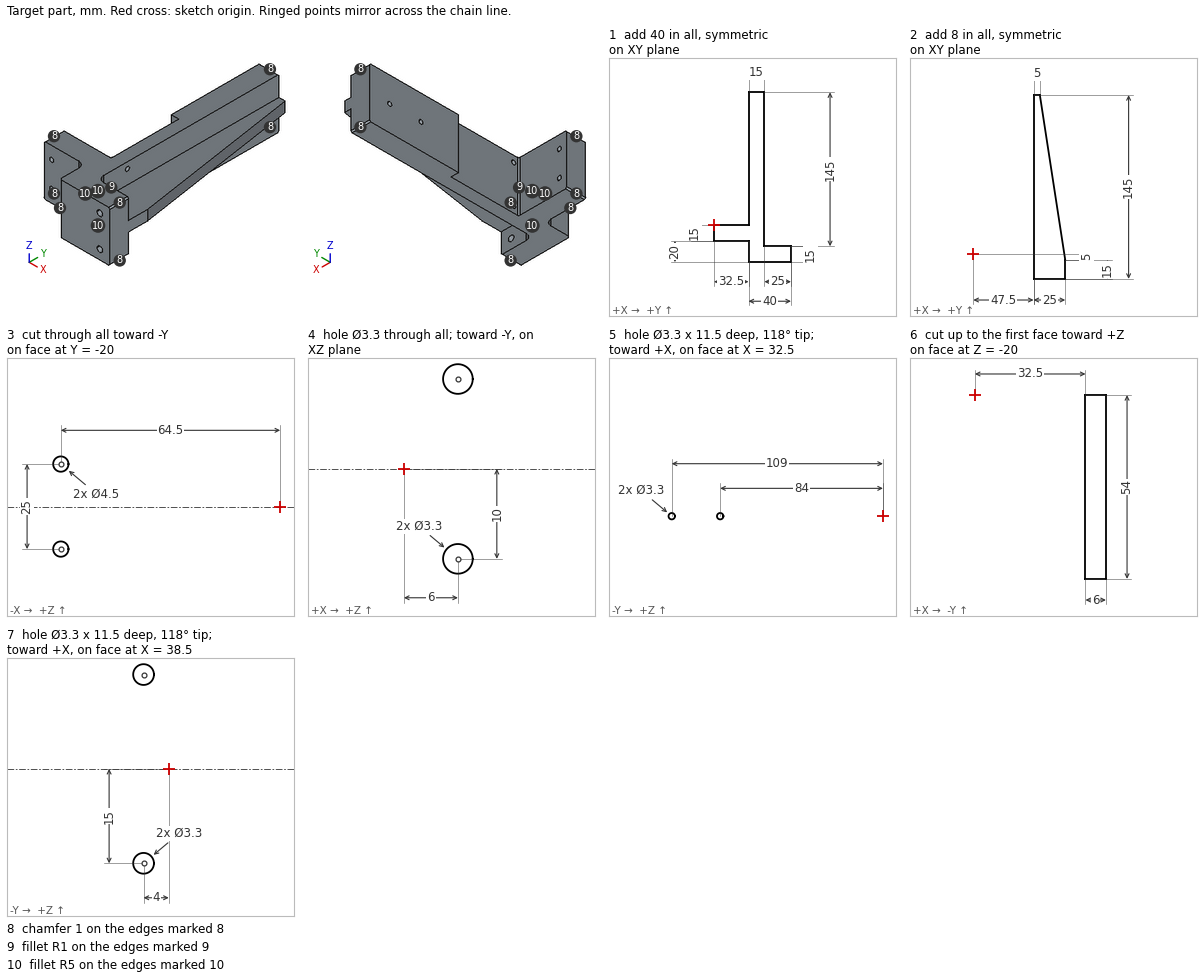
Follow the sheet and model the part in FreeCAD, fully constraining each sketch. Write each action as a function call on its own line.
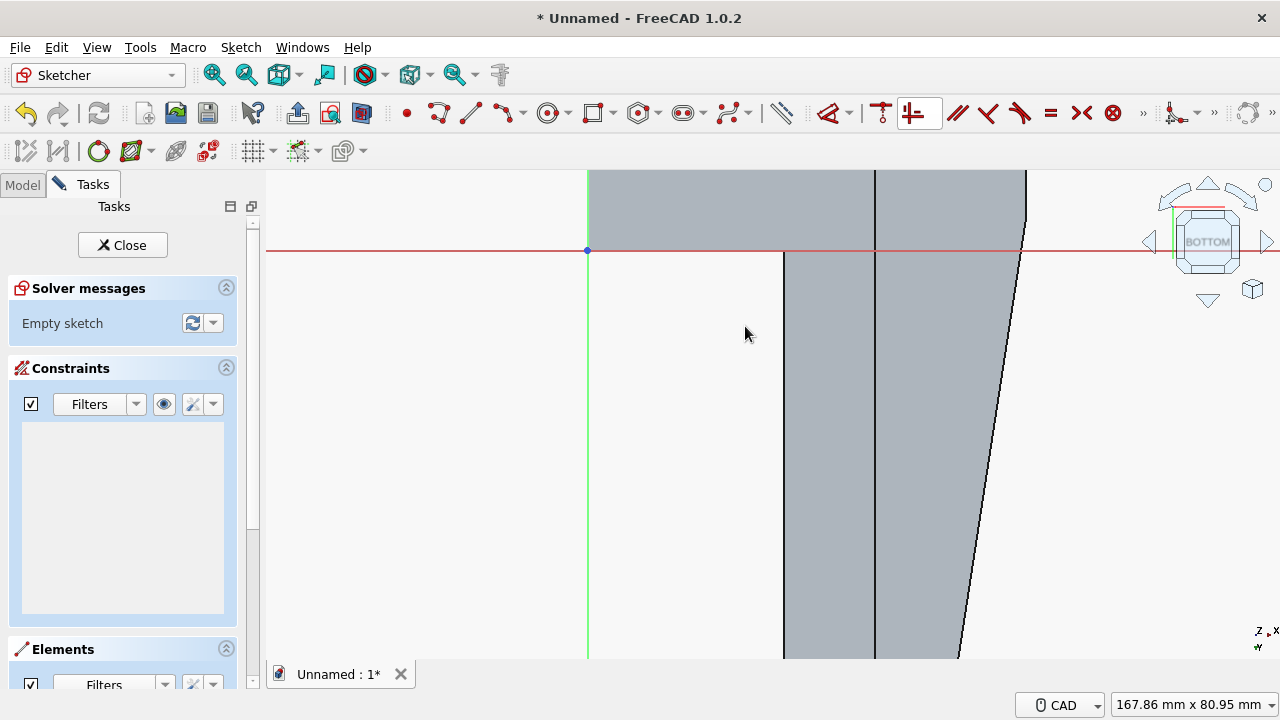
key(g)
key(r)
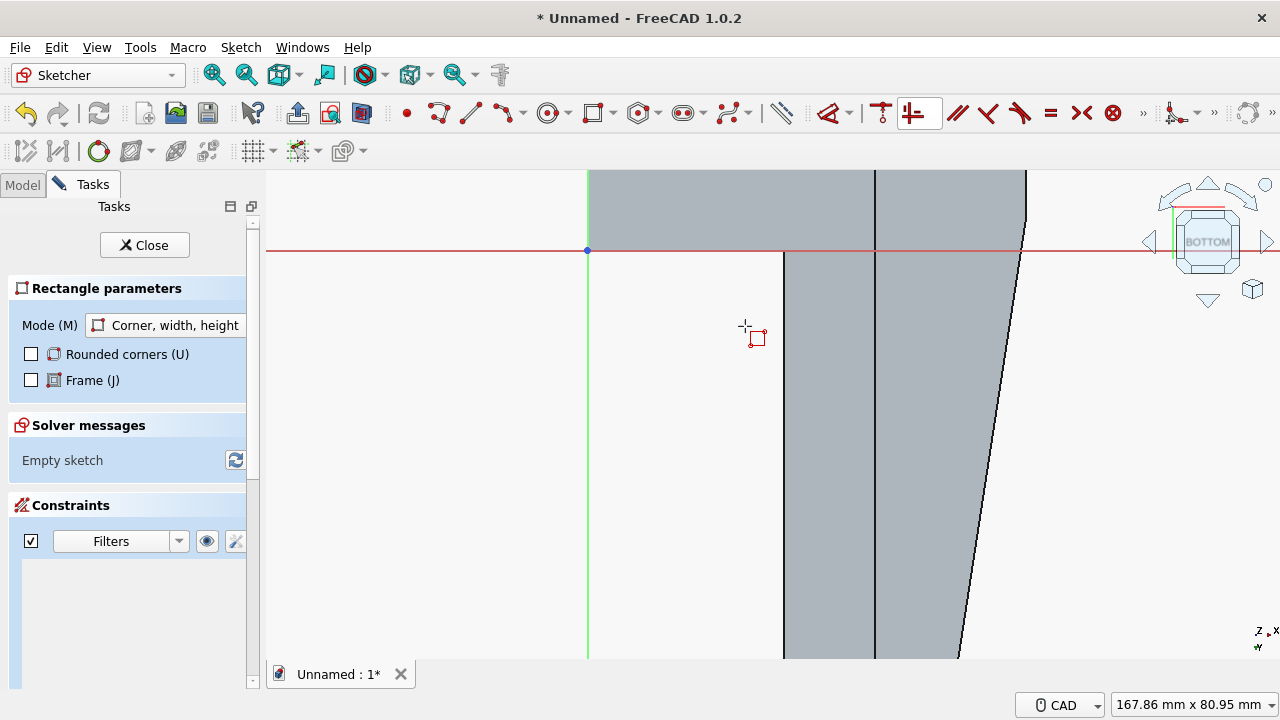
click(784, 251)
click(820, 577)
key(Escape)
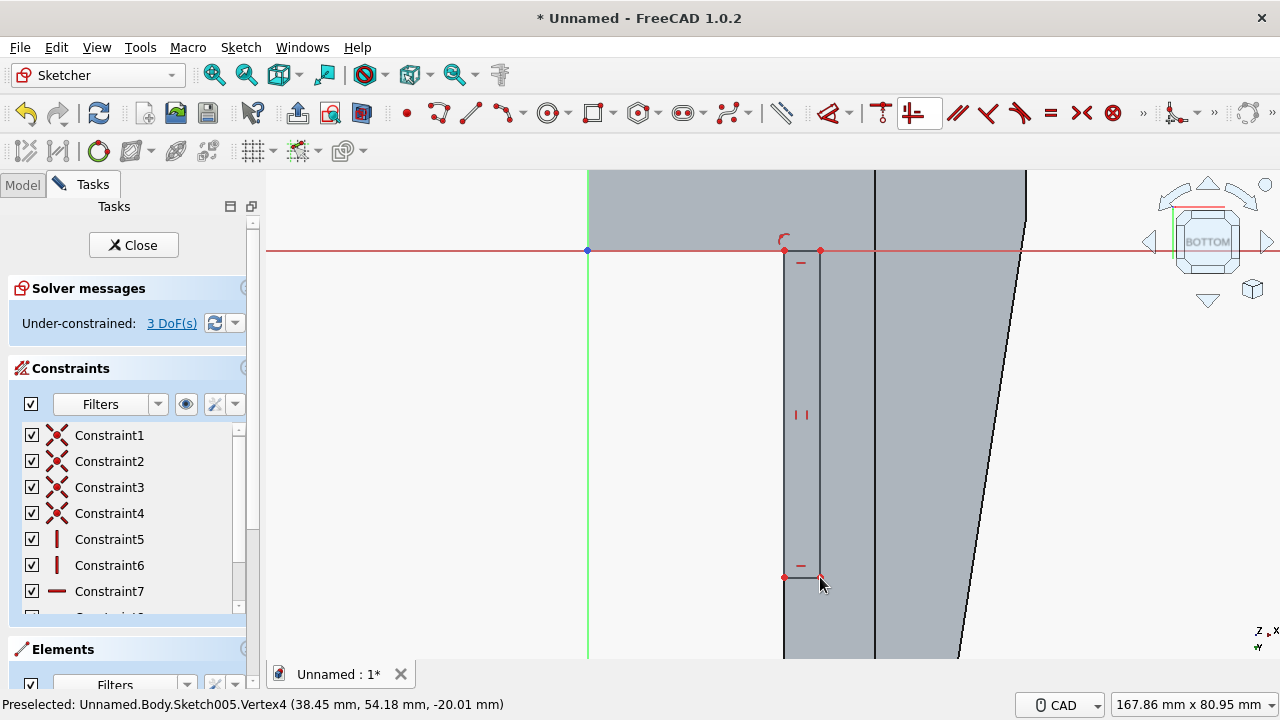
click(828, 114)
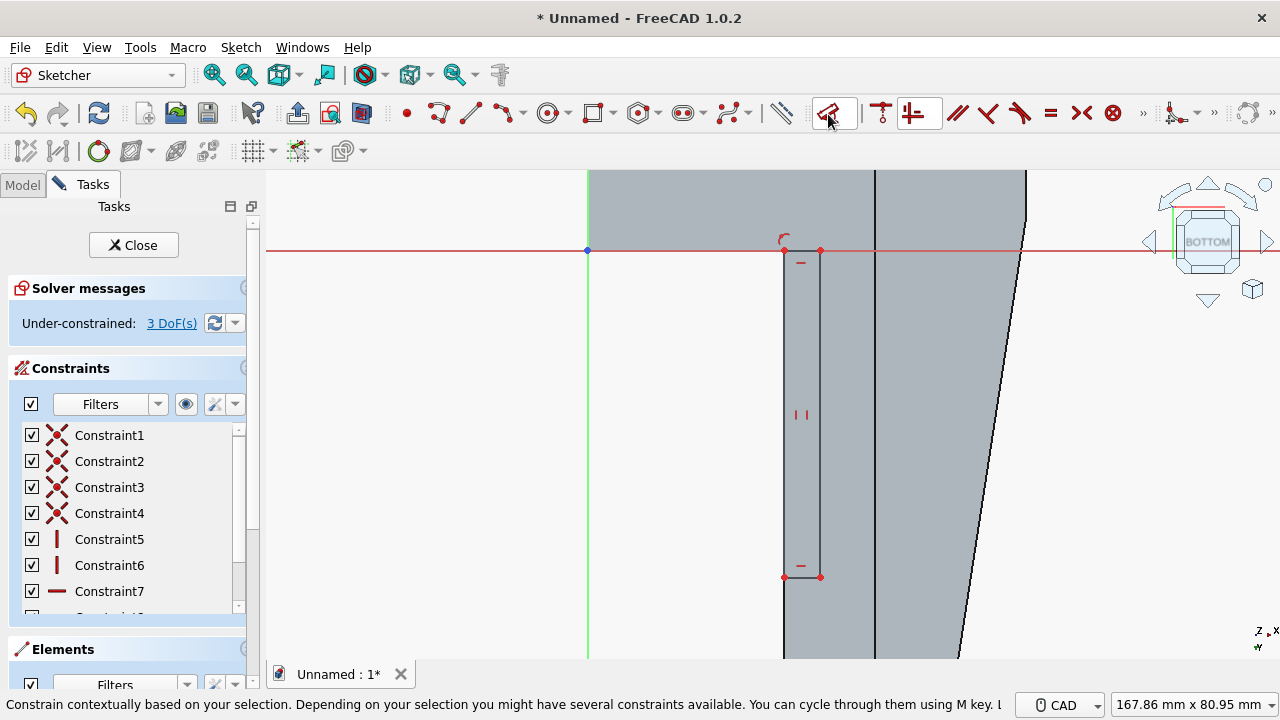
scroll(795, 578, up, 2)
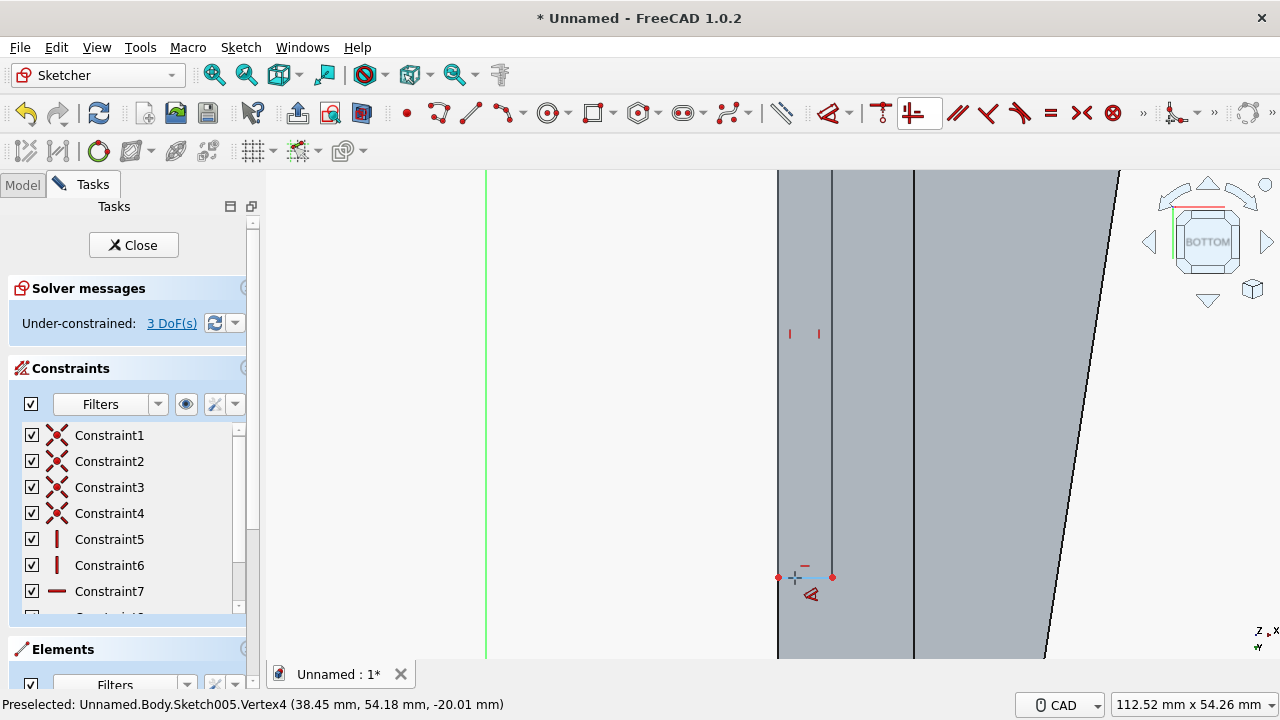
click(794, 578)
click(805, 612)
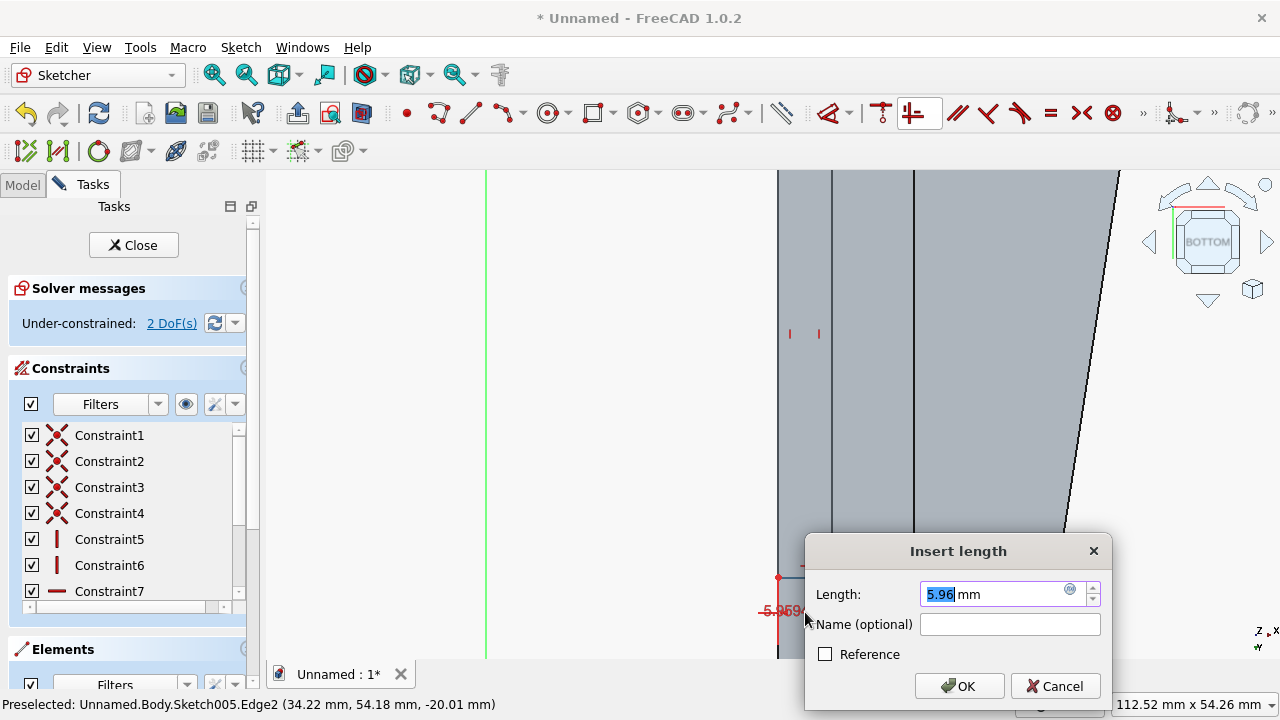
text(6)
key(Return)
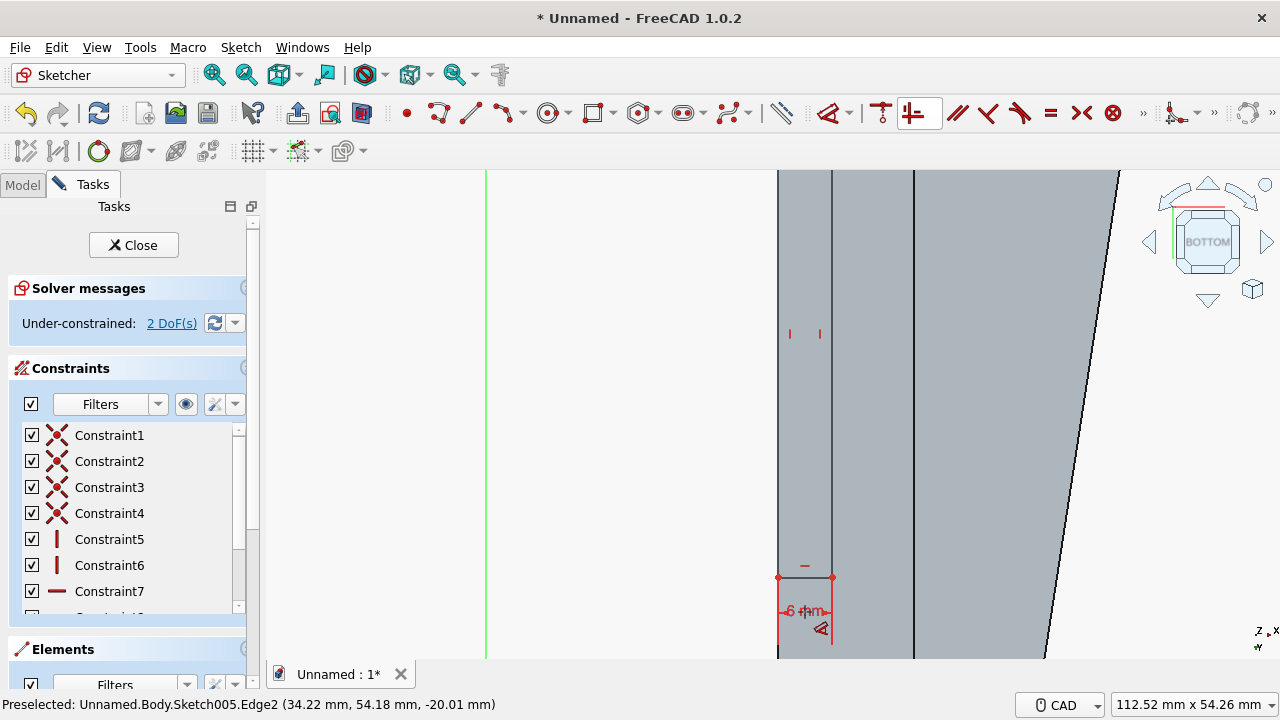
click(778, 236)
click(812, 388)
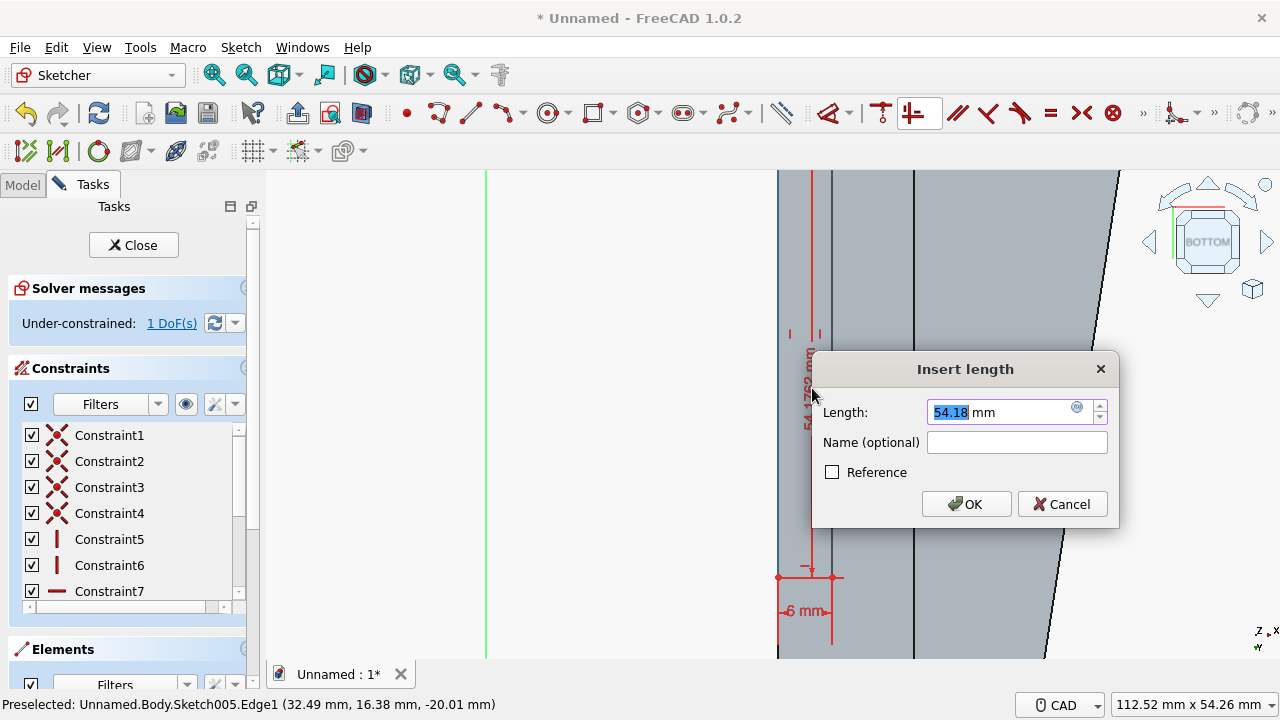
text(54)
key(Return)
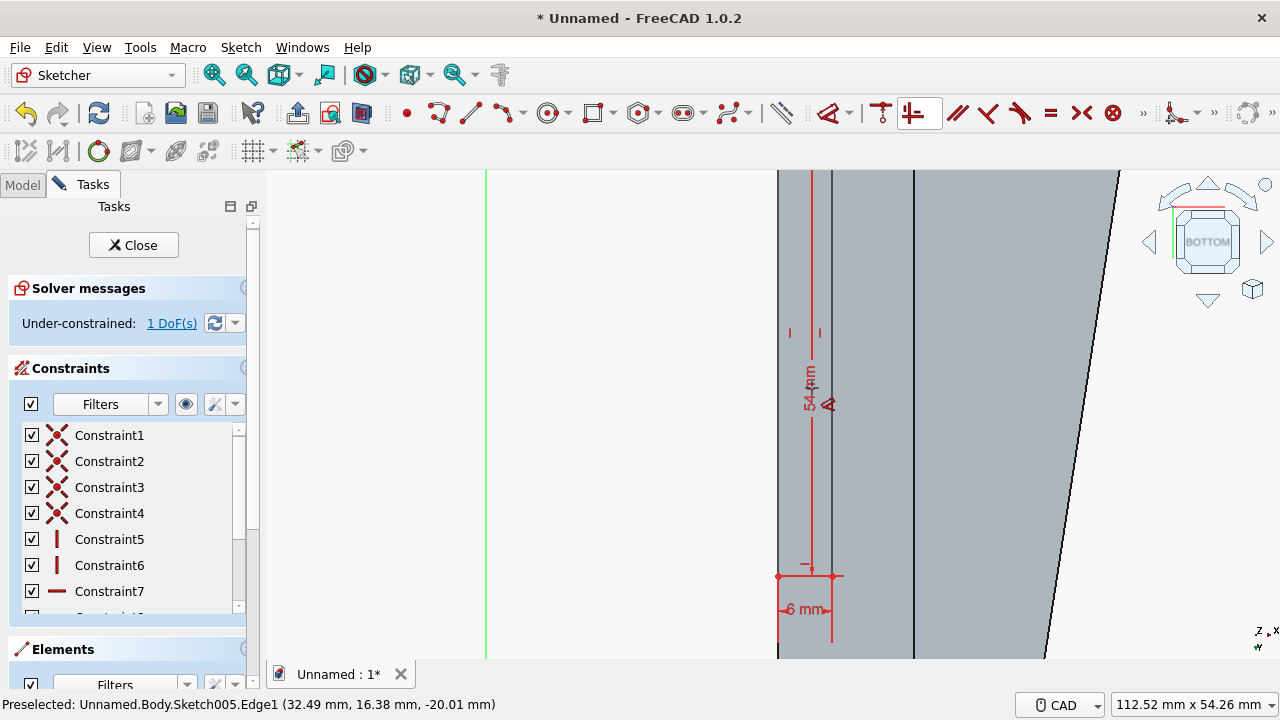
scroll(797, 581, down, 2)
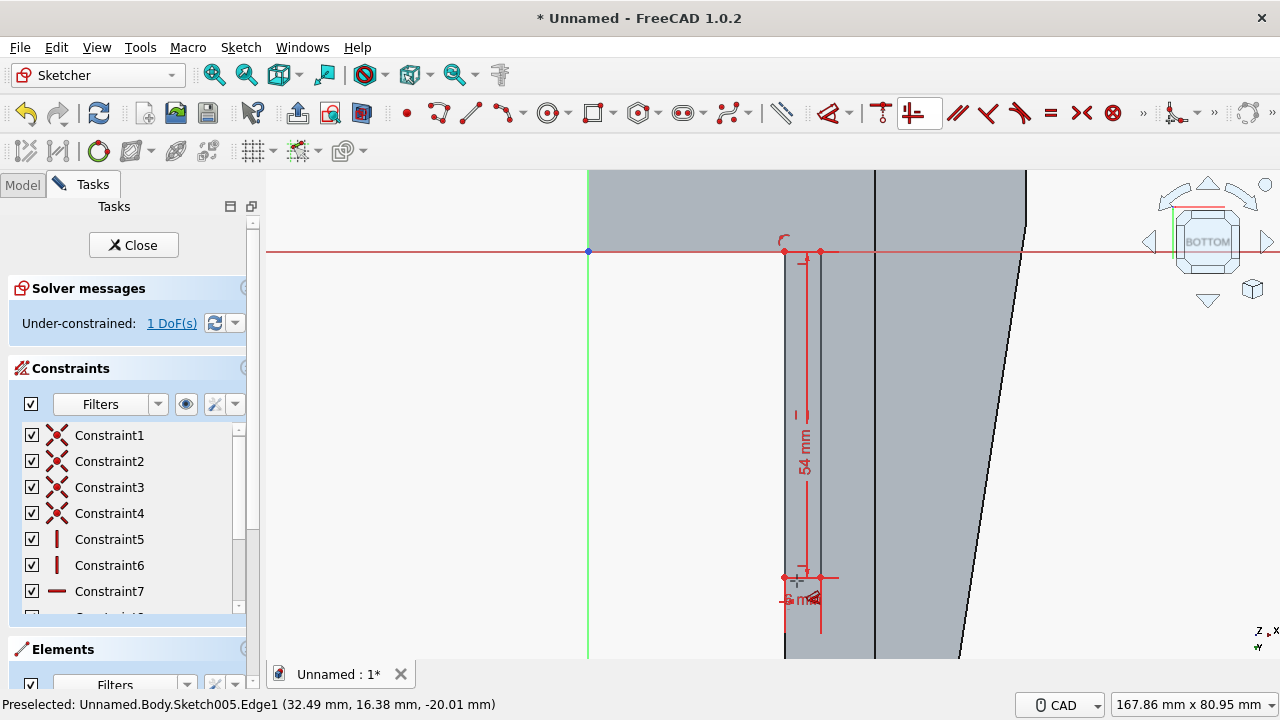
click(785, 252)
click(687, 218)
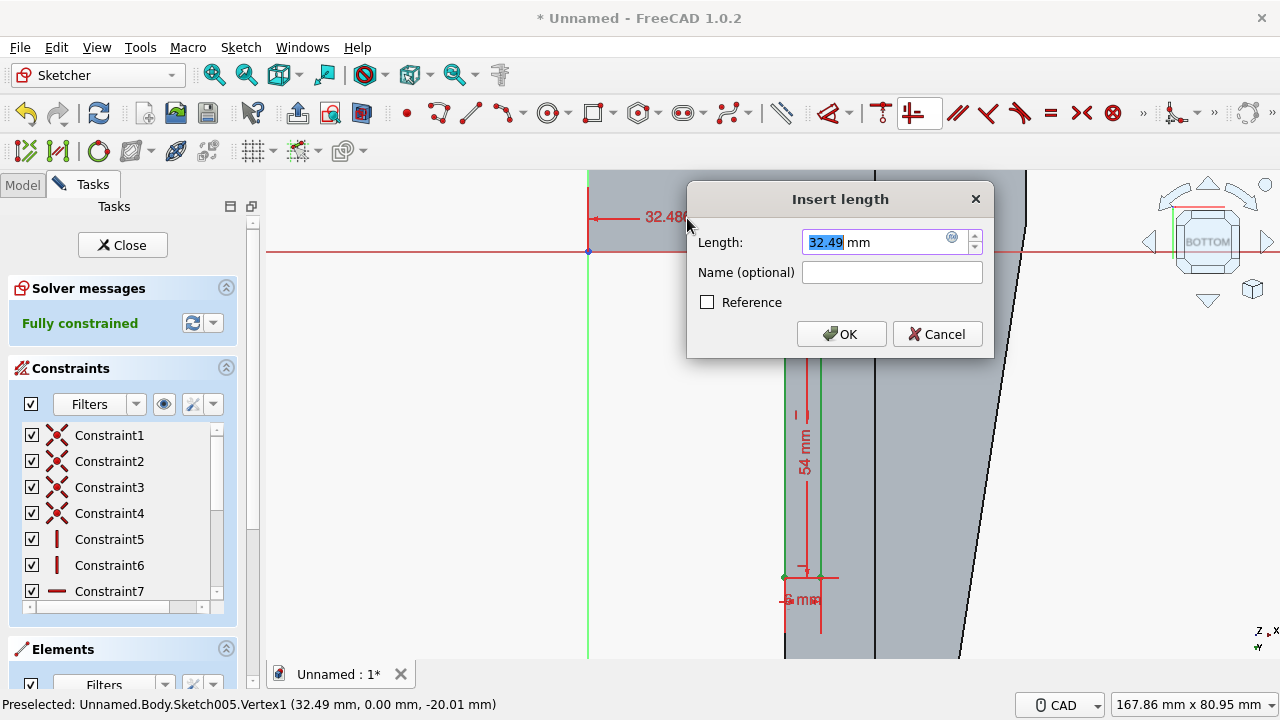
text(32.5)
key(Return)
key(Escape)